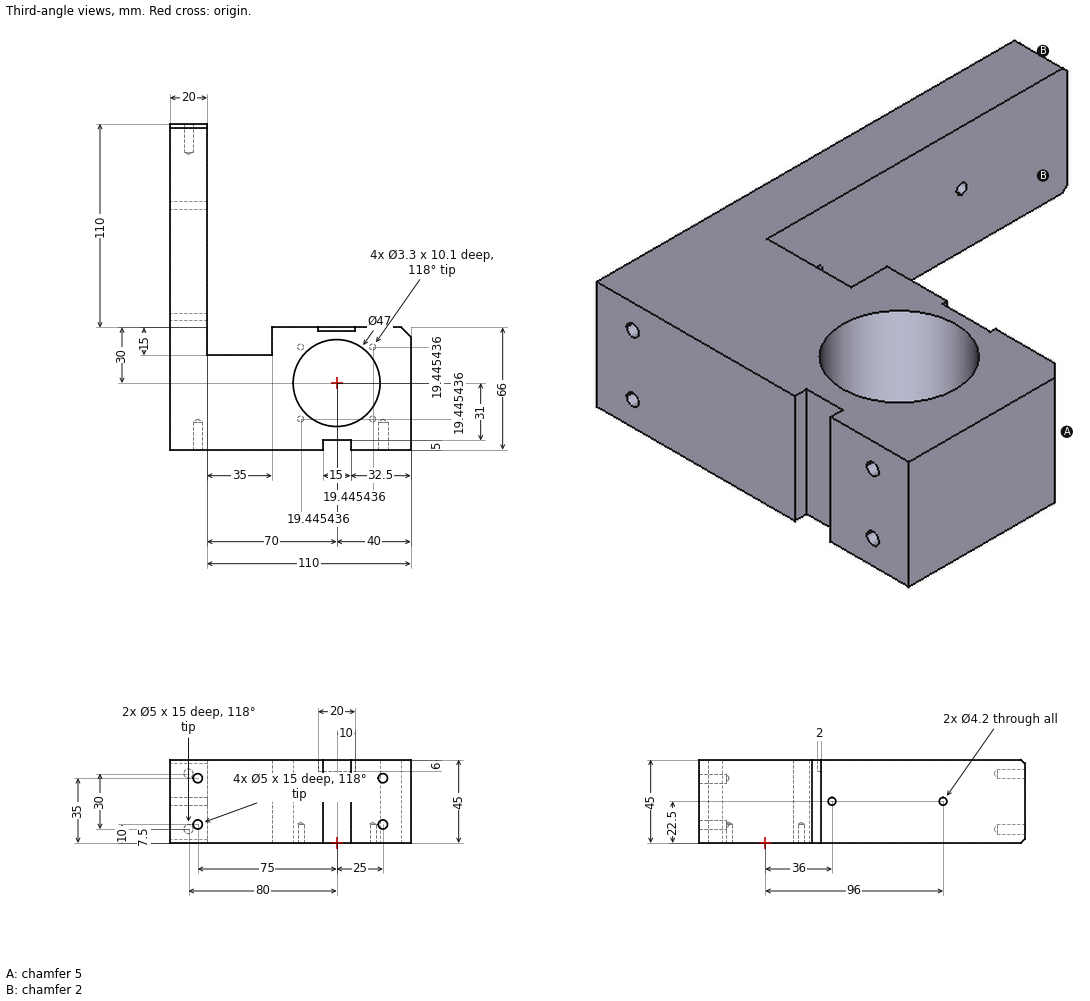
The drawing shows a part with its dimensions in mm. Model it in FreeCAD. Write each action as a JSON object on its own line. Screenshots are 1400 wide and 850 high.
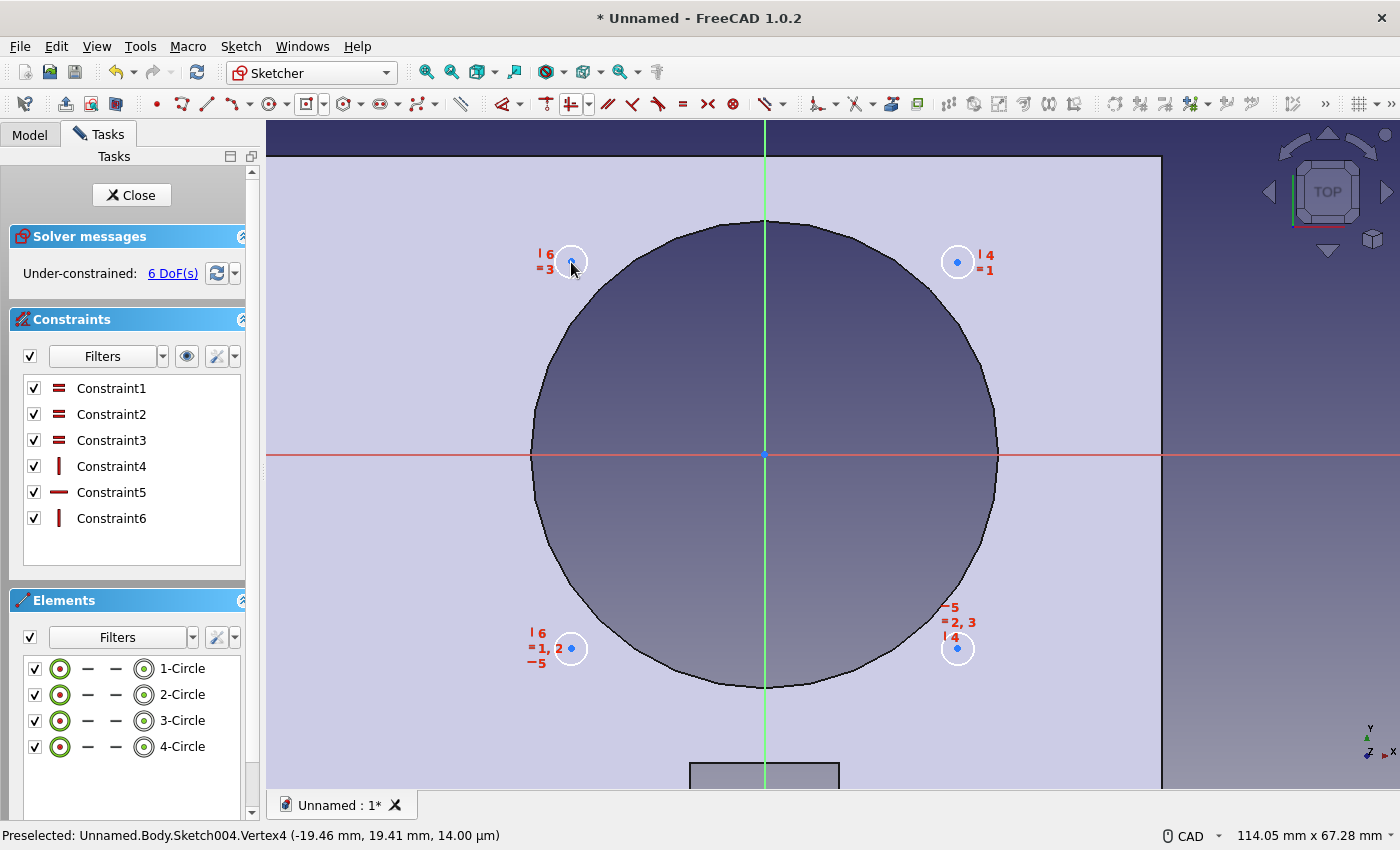
{"action": "left_click", "coordinate": [958, 262]}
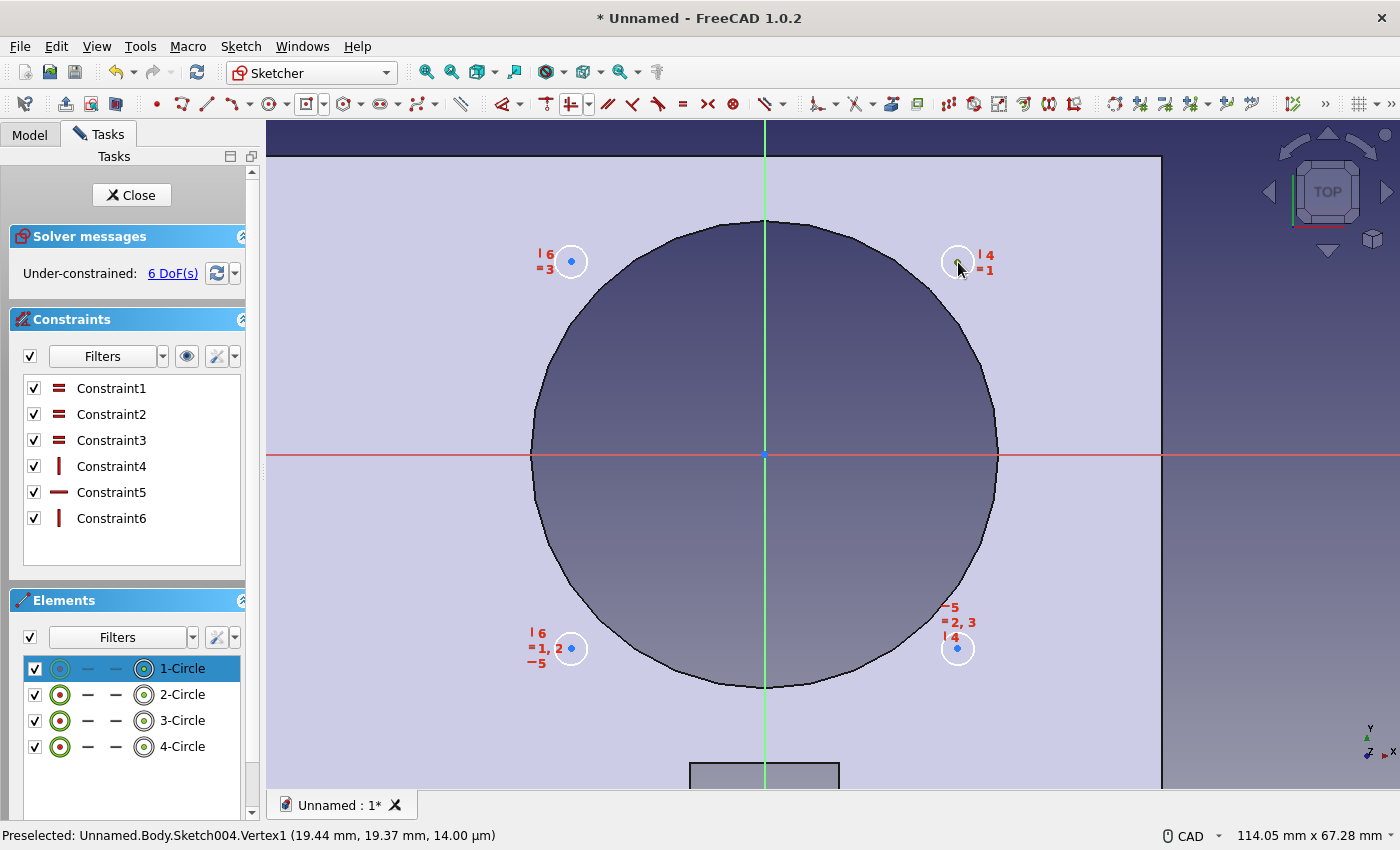
{"action": "left_click", "coordinate": [571, 262]}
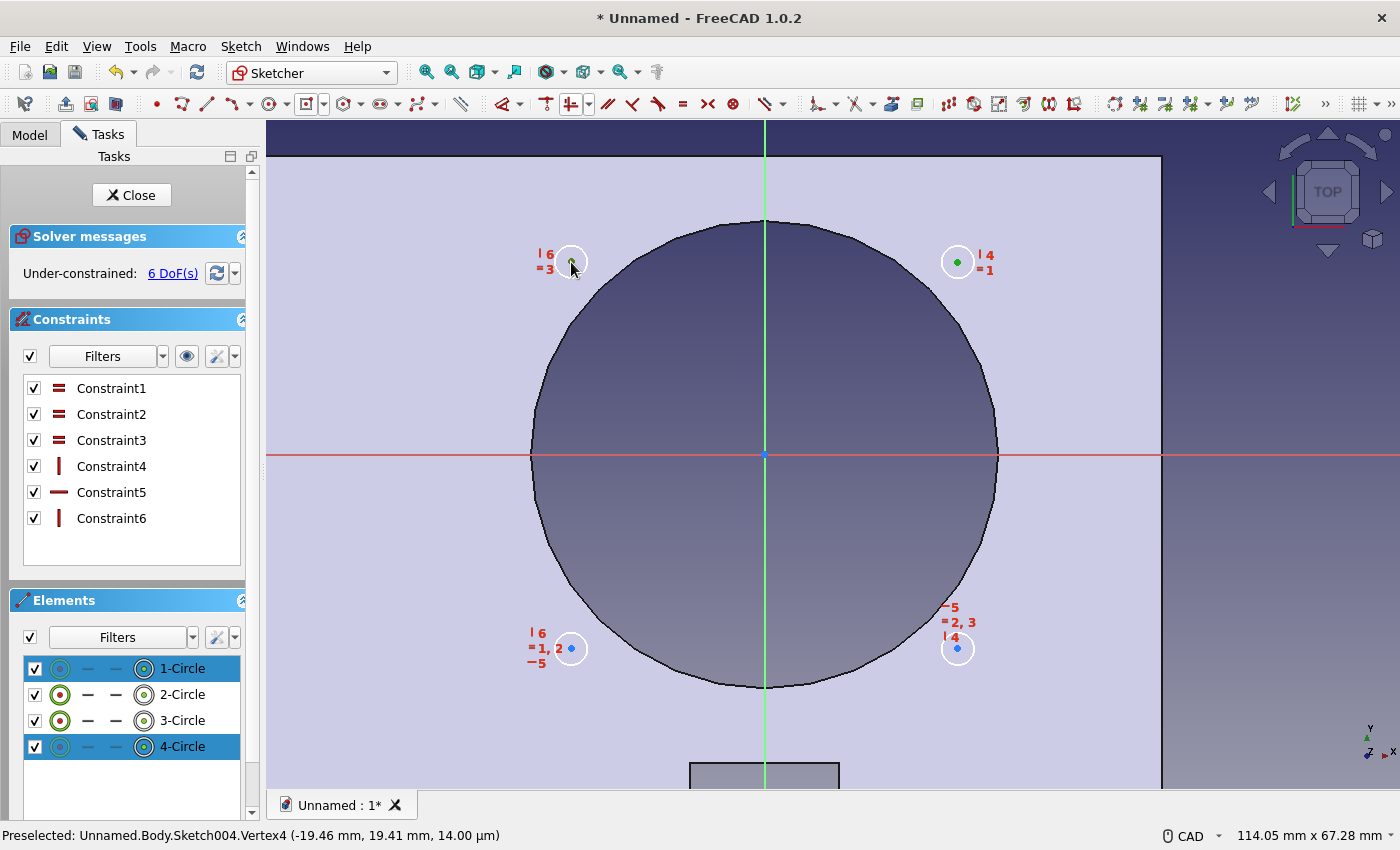
{"action": "key", "text": "h"}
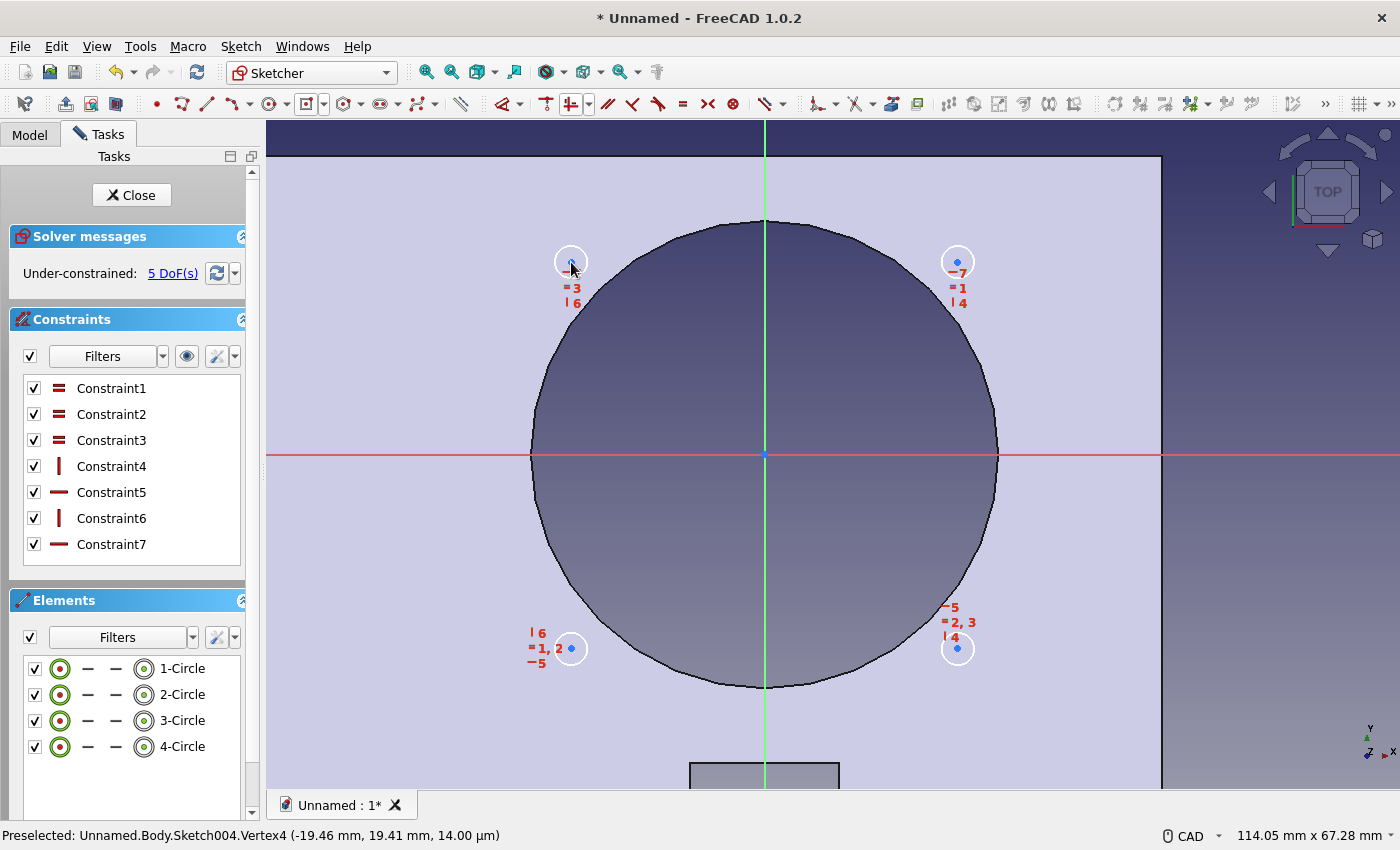
{"action": "left_click", "coordinate": [502, 104]}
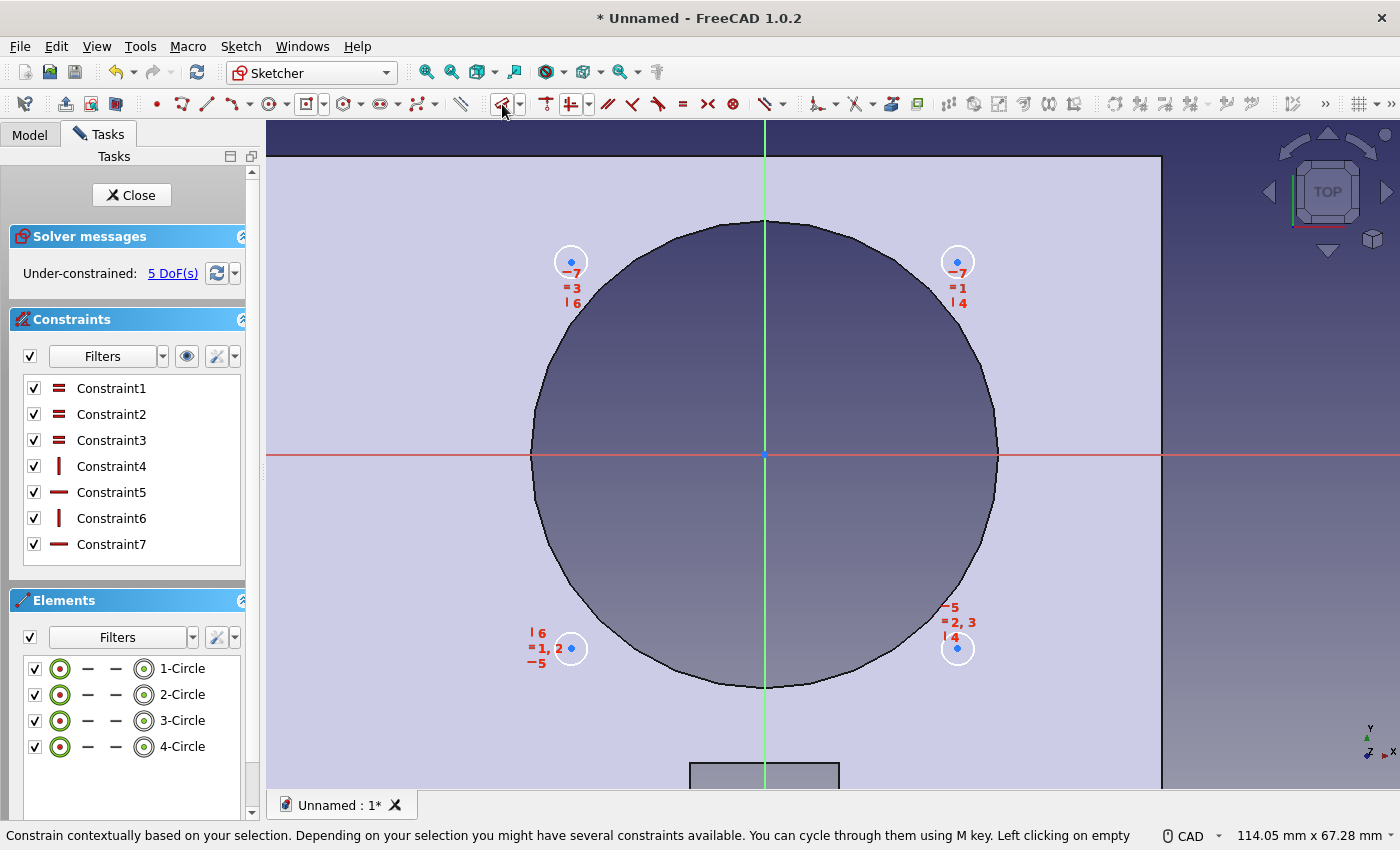
{"action": "left_click", "coordinate": [969, 251]}
{"action": "left_click", "coordinate": [992, 228]}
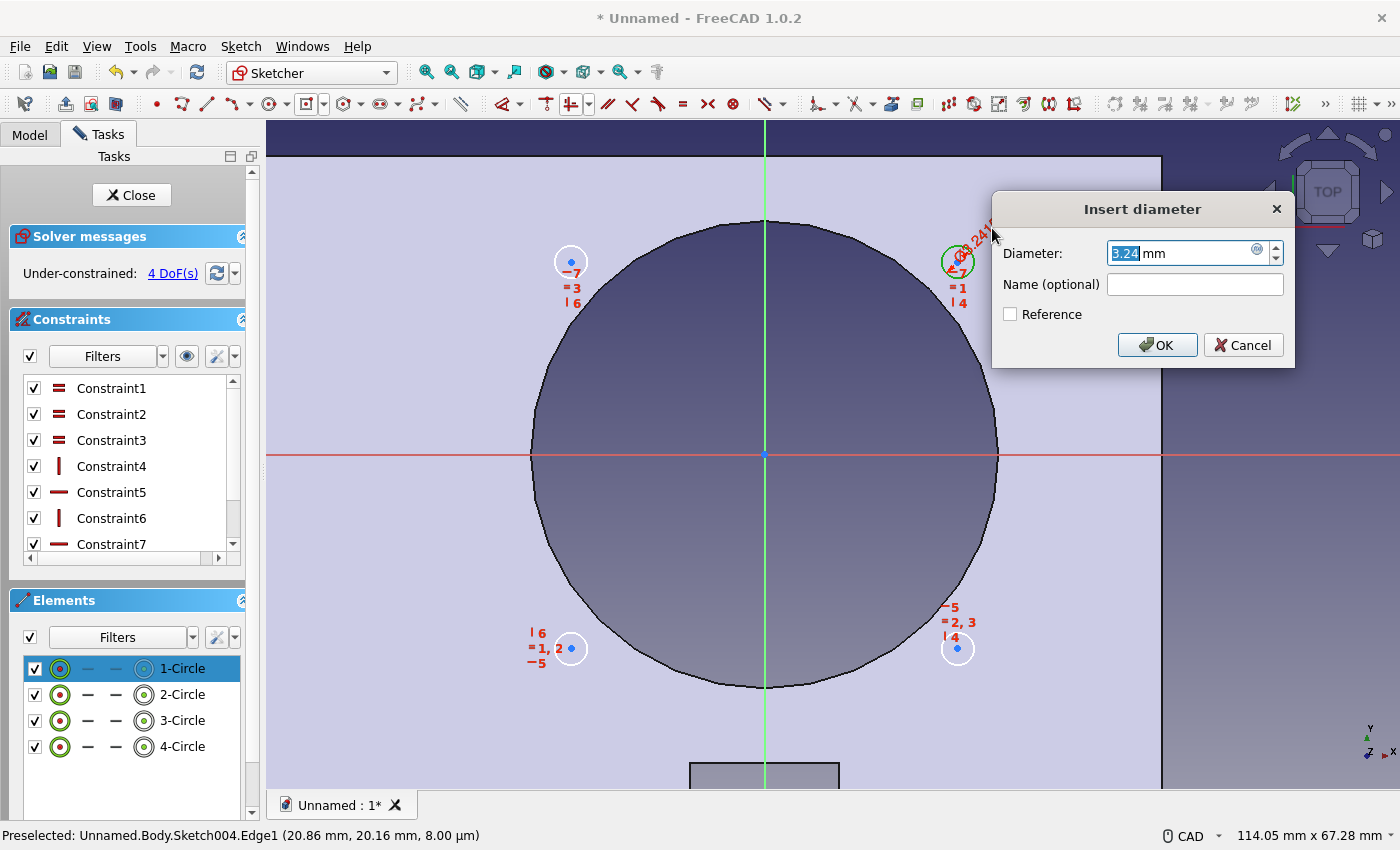
{"action": "type", "text": "3.3"}
{"action": "key", "text": "Return"}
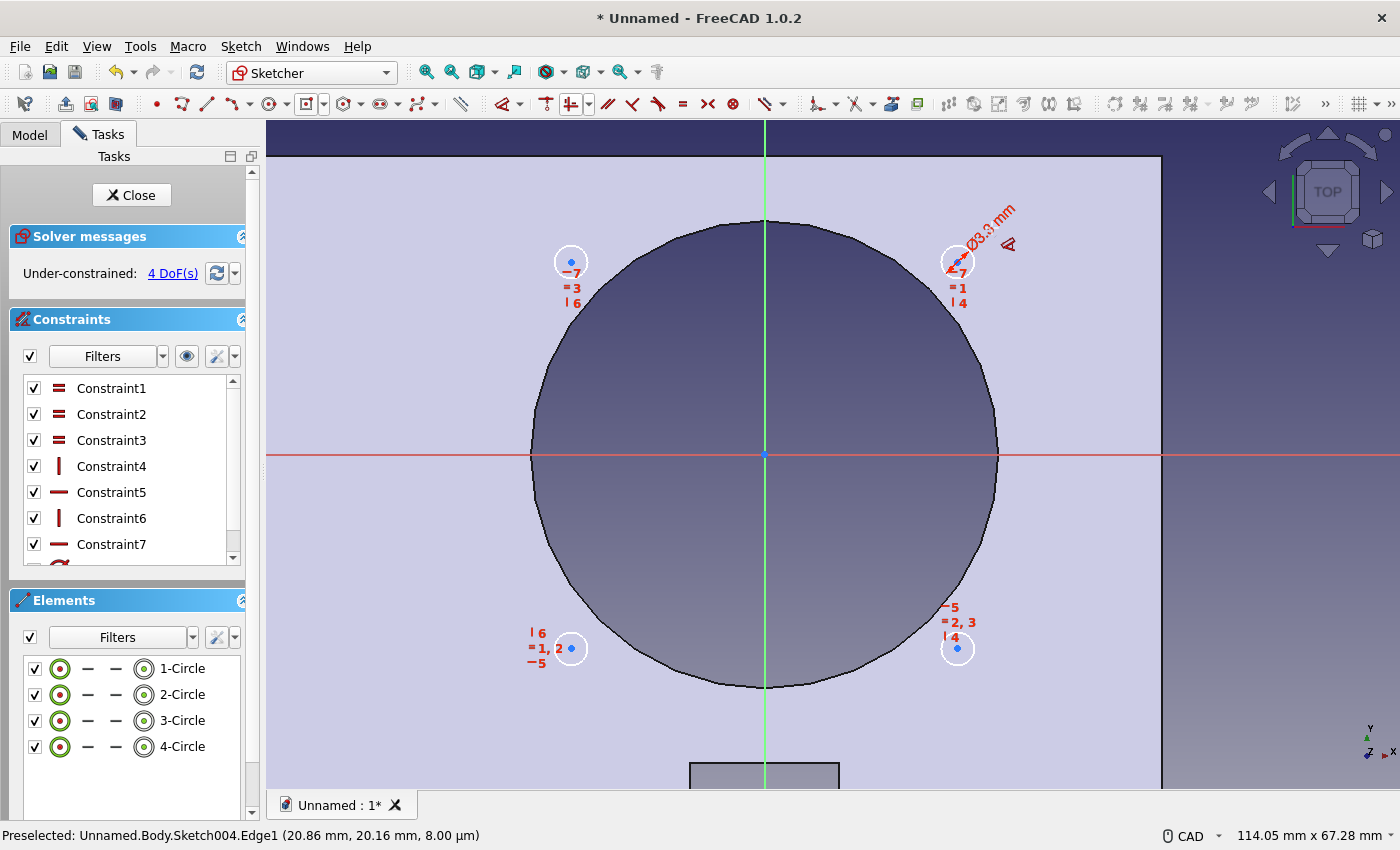
{"action": "left_click", "coordinate": [958, 262]}
{"action": "left_click", "coordinate": [861, 228]}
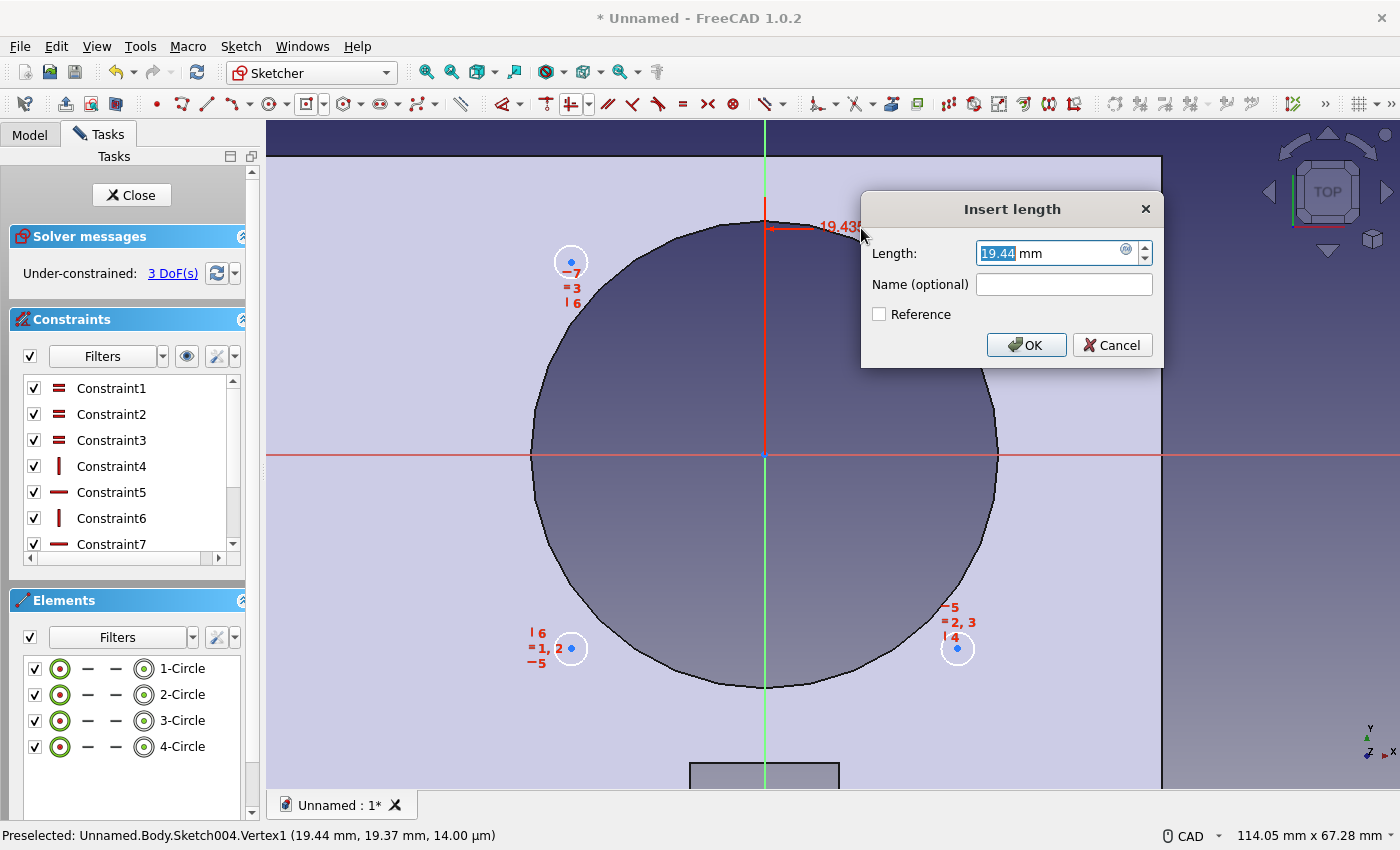
{"action": "type", "text": "19.445436"}
{"action": "key", "text": "Return"}